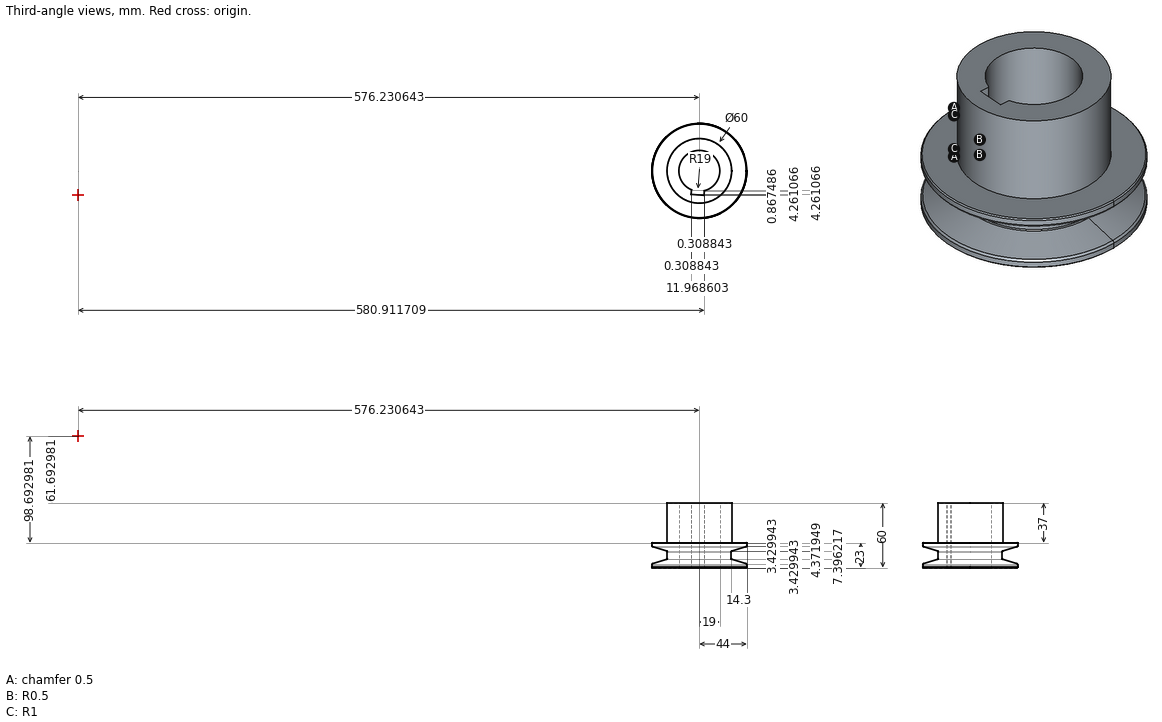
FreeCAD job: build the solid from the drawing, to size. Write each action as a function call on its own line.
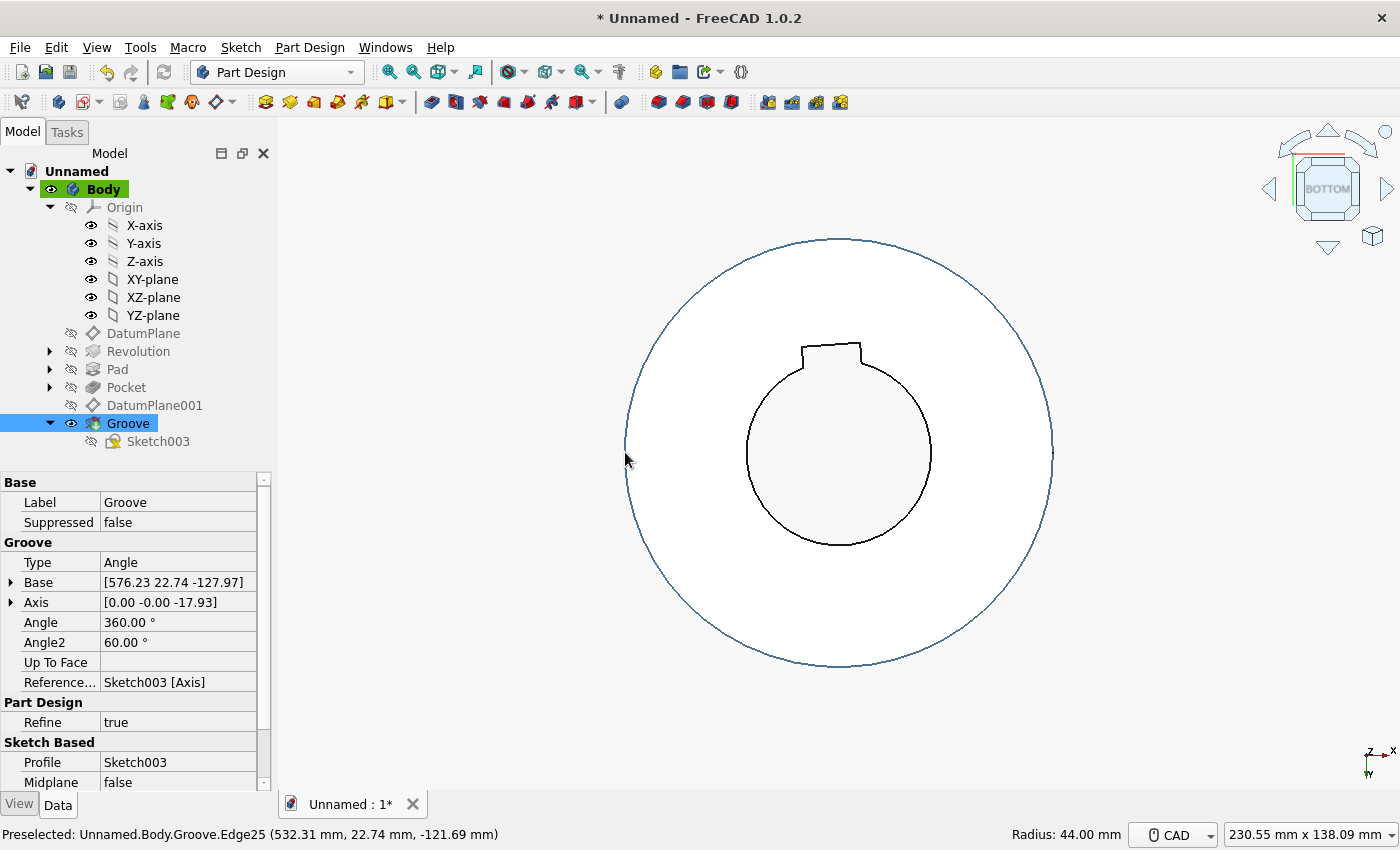
key(0)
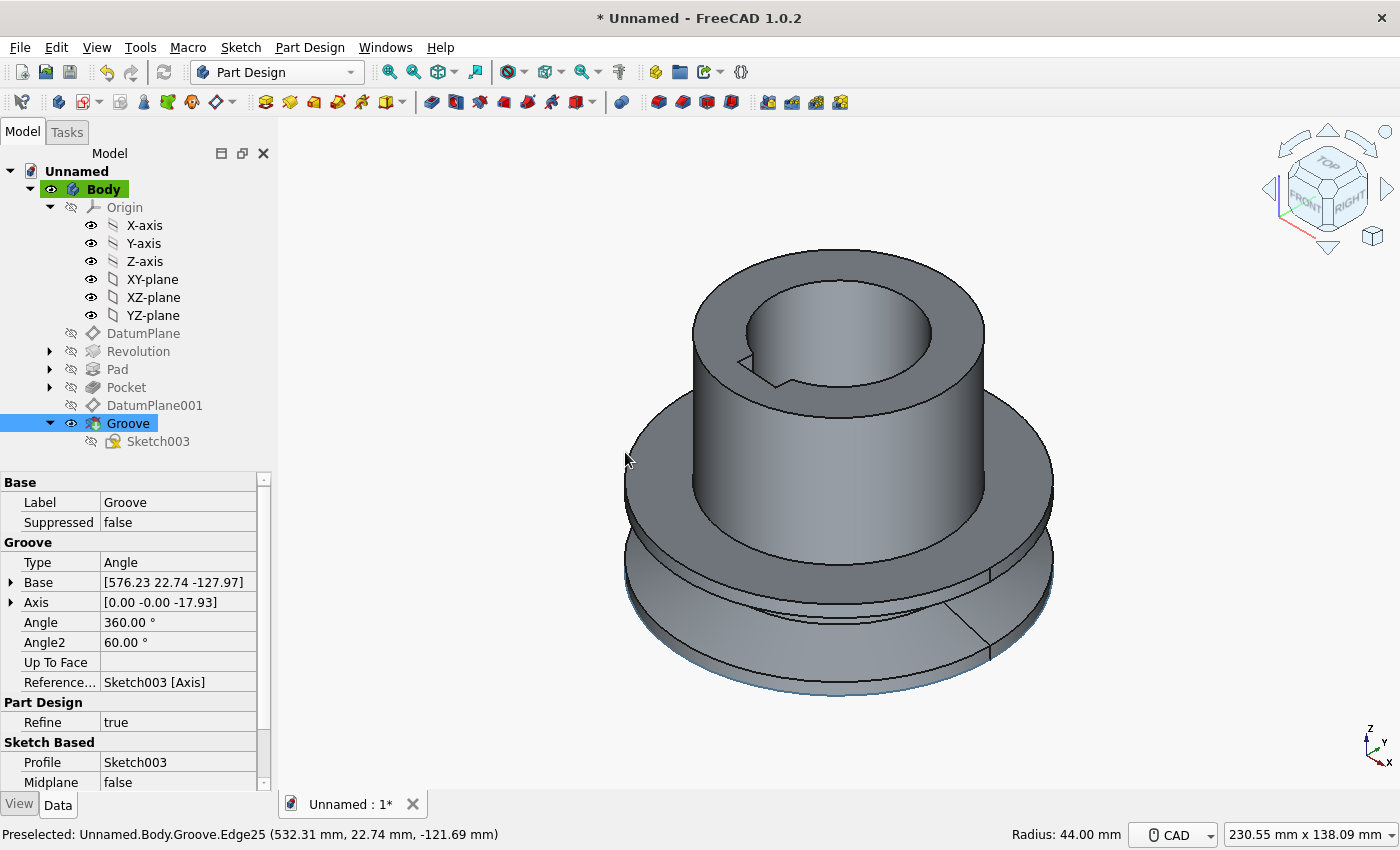
click(627, 460, ctrl)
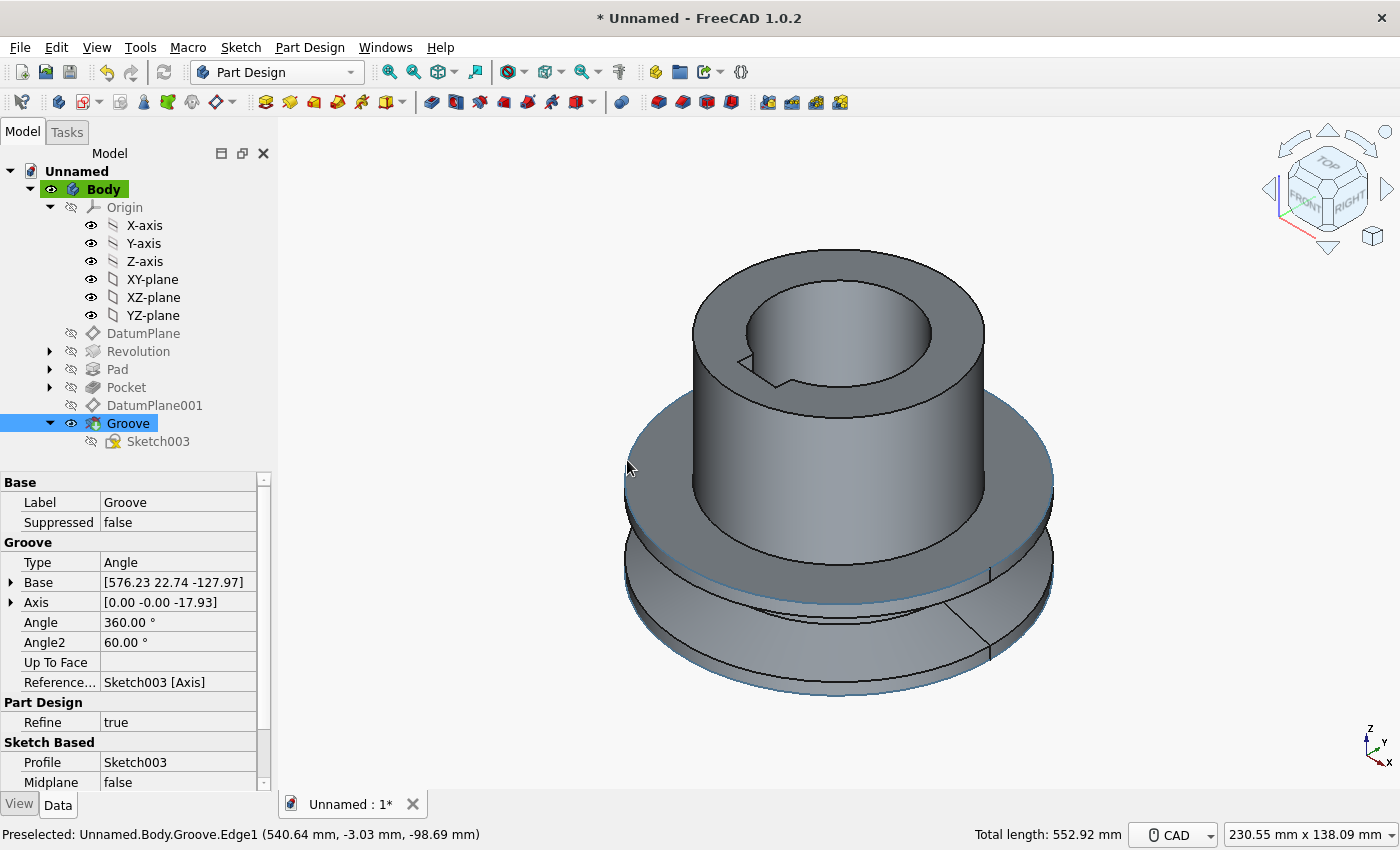
click(684, 102)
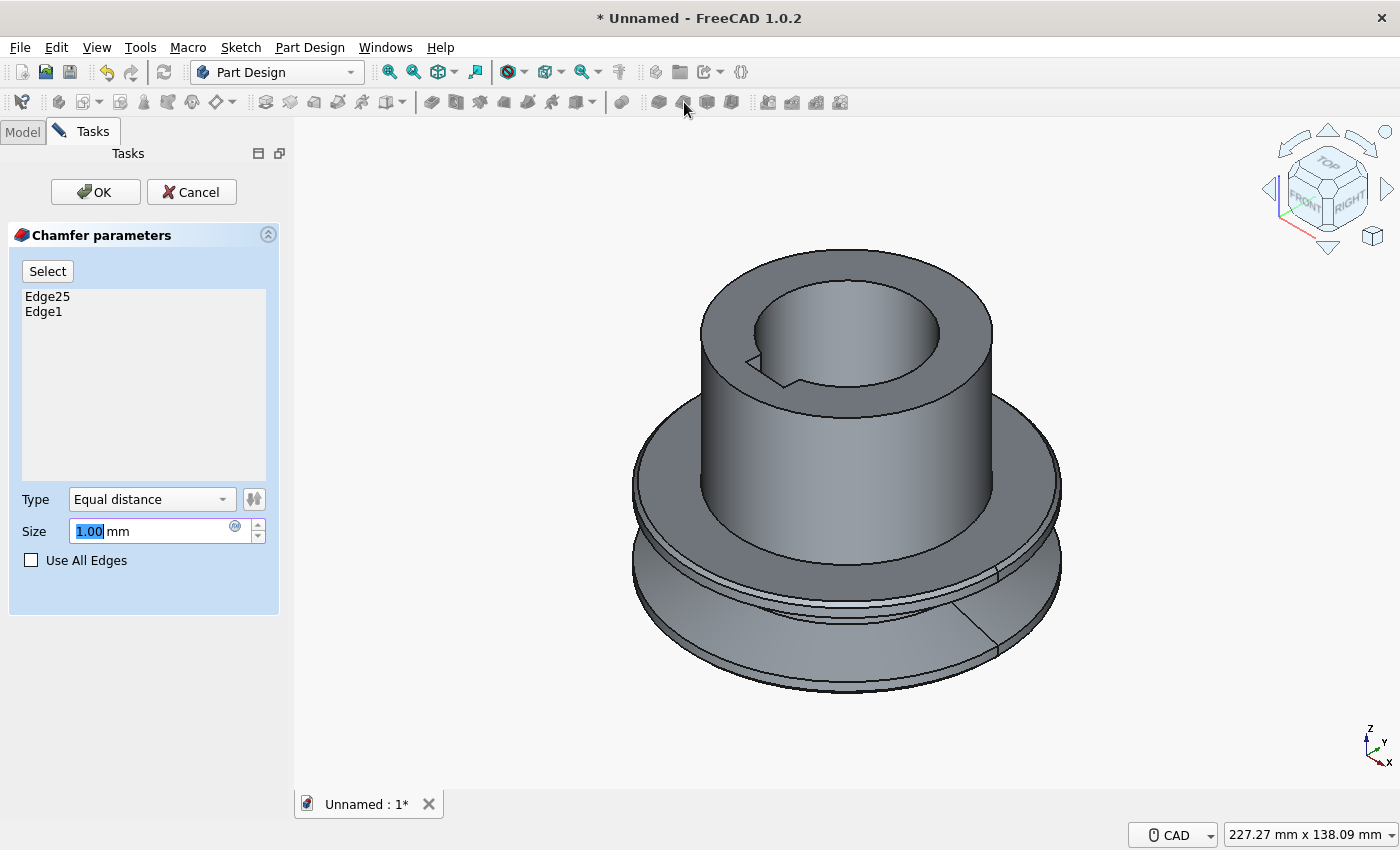
text(0.5)
key(Tab)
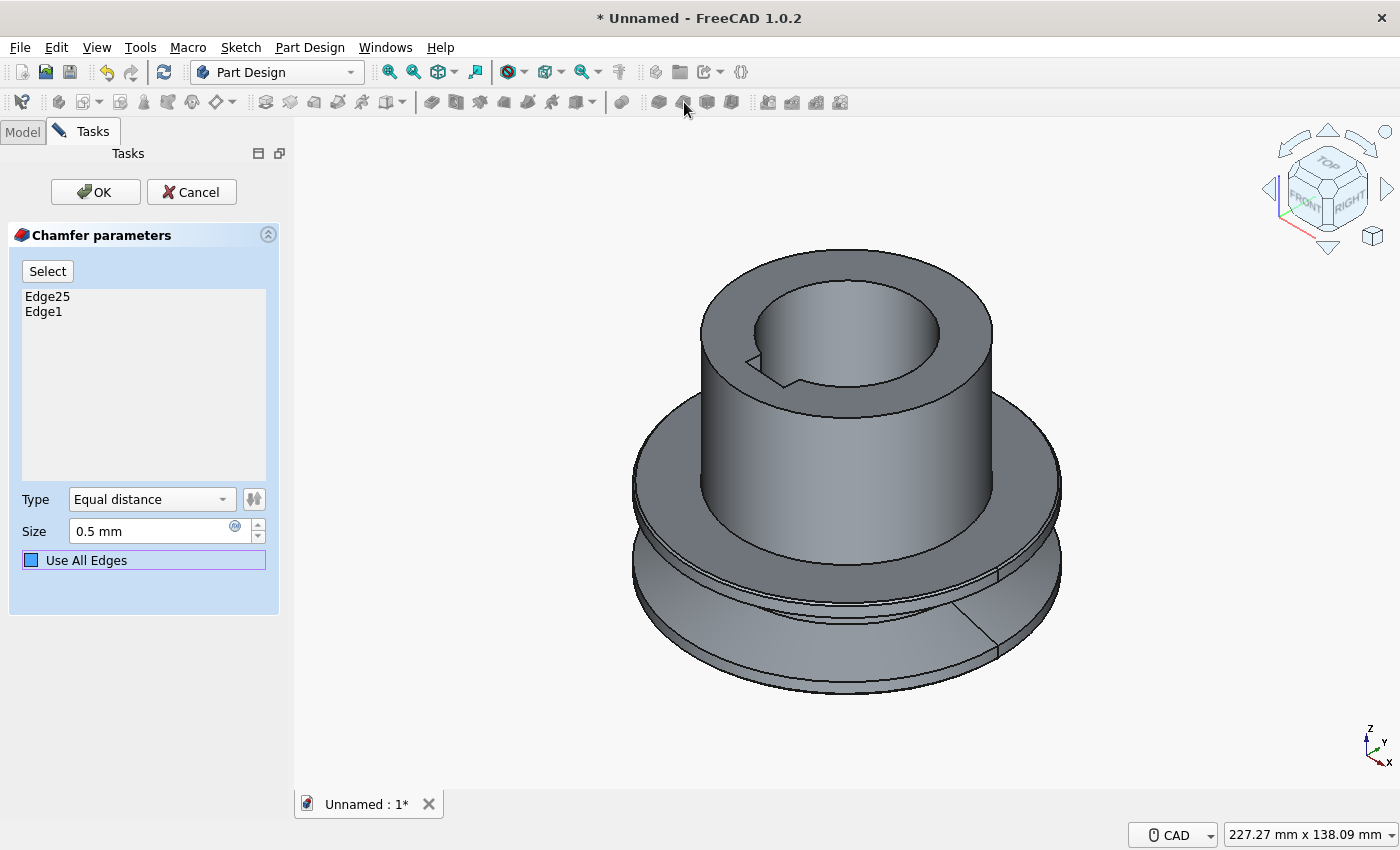
click(96, 192)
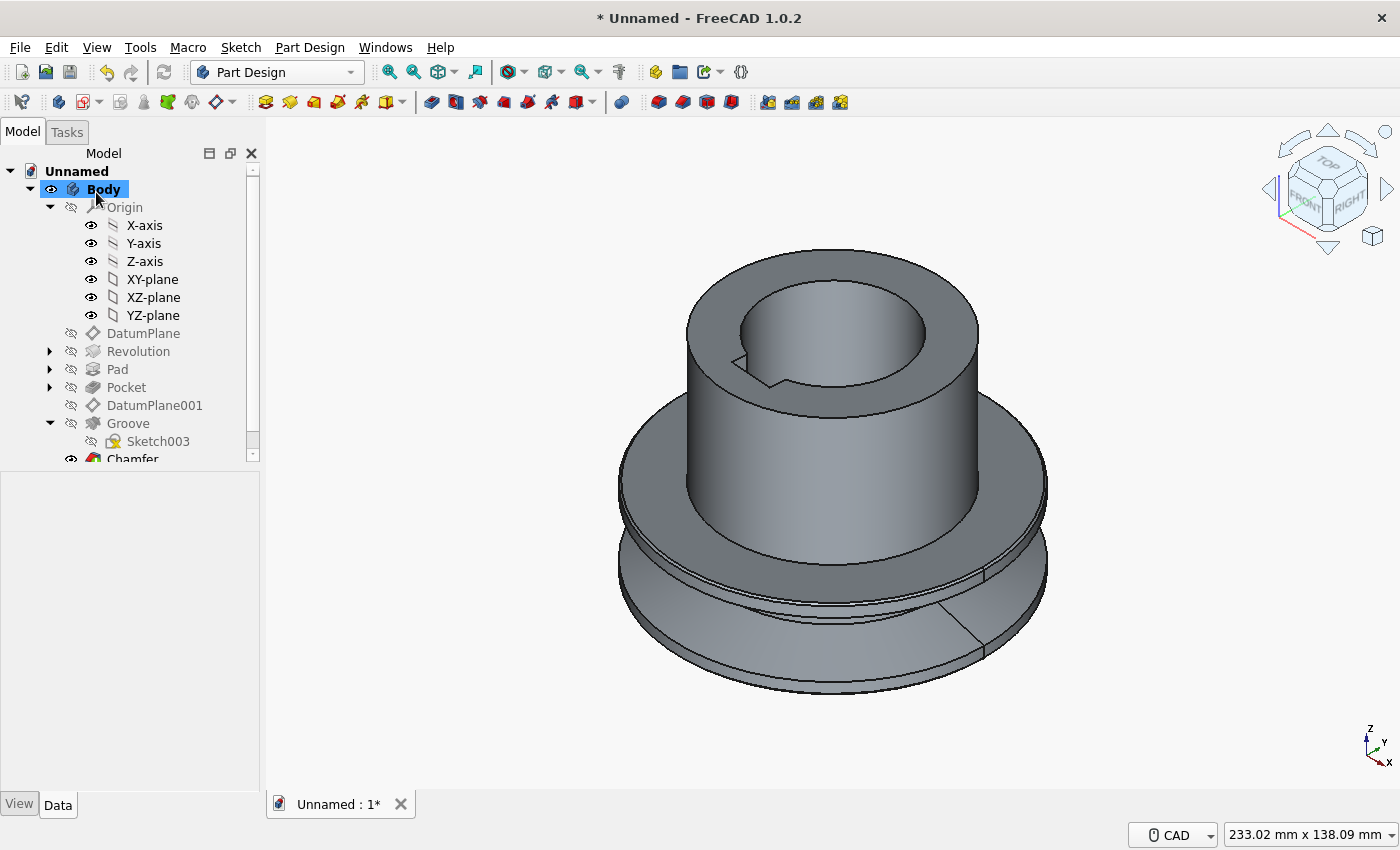
key(2)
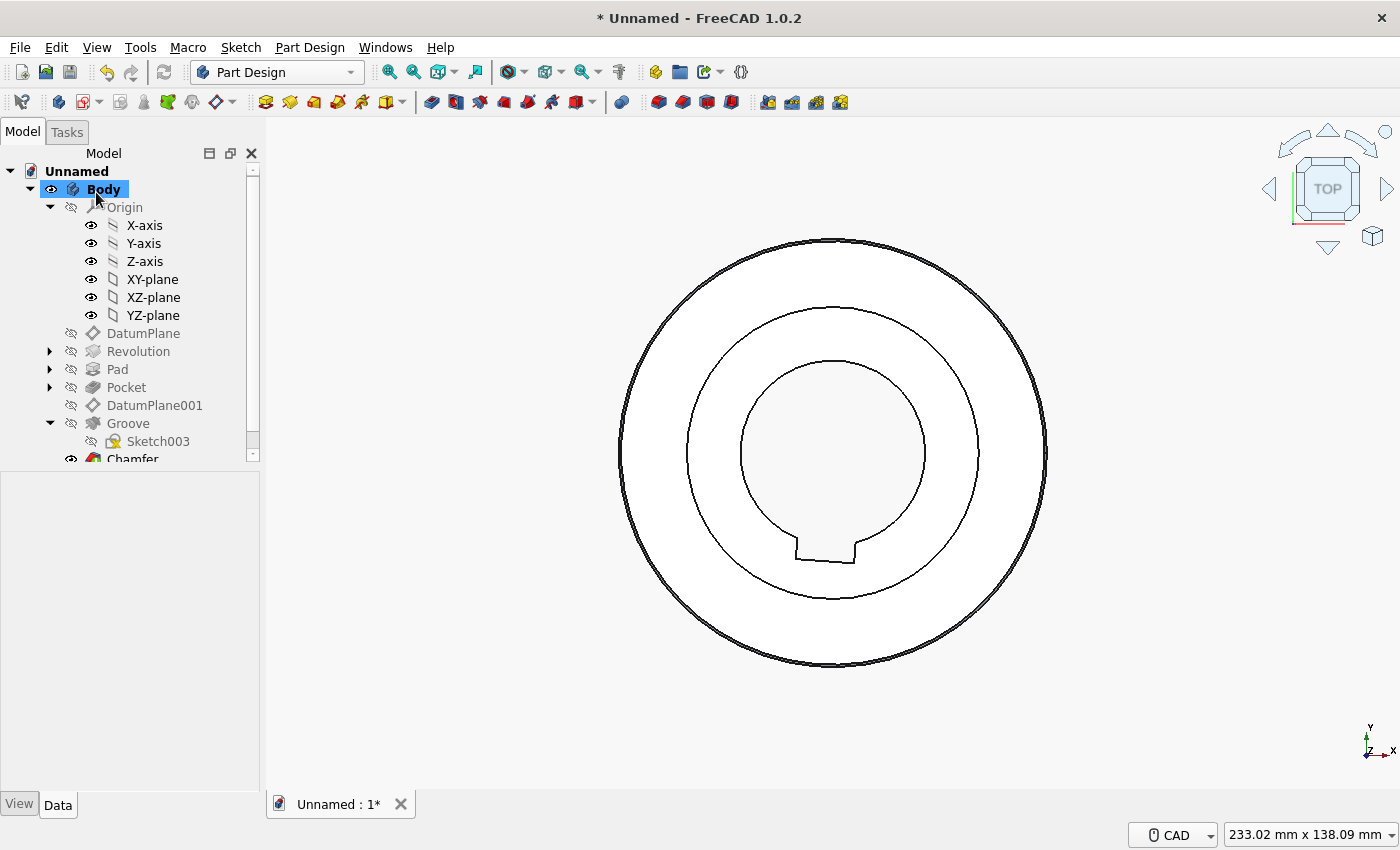
key(0)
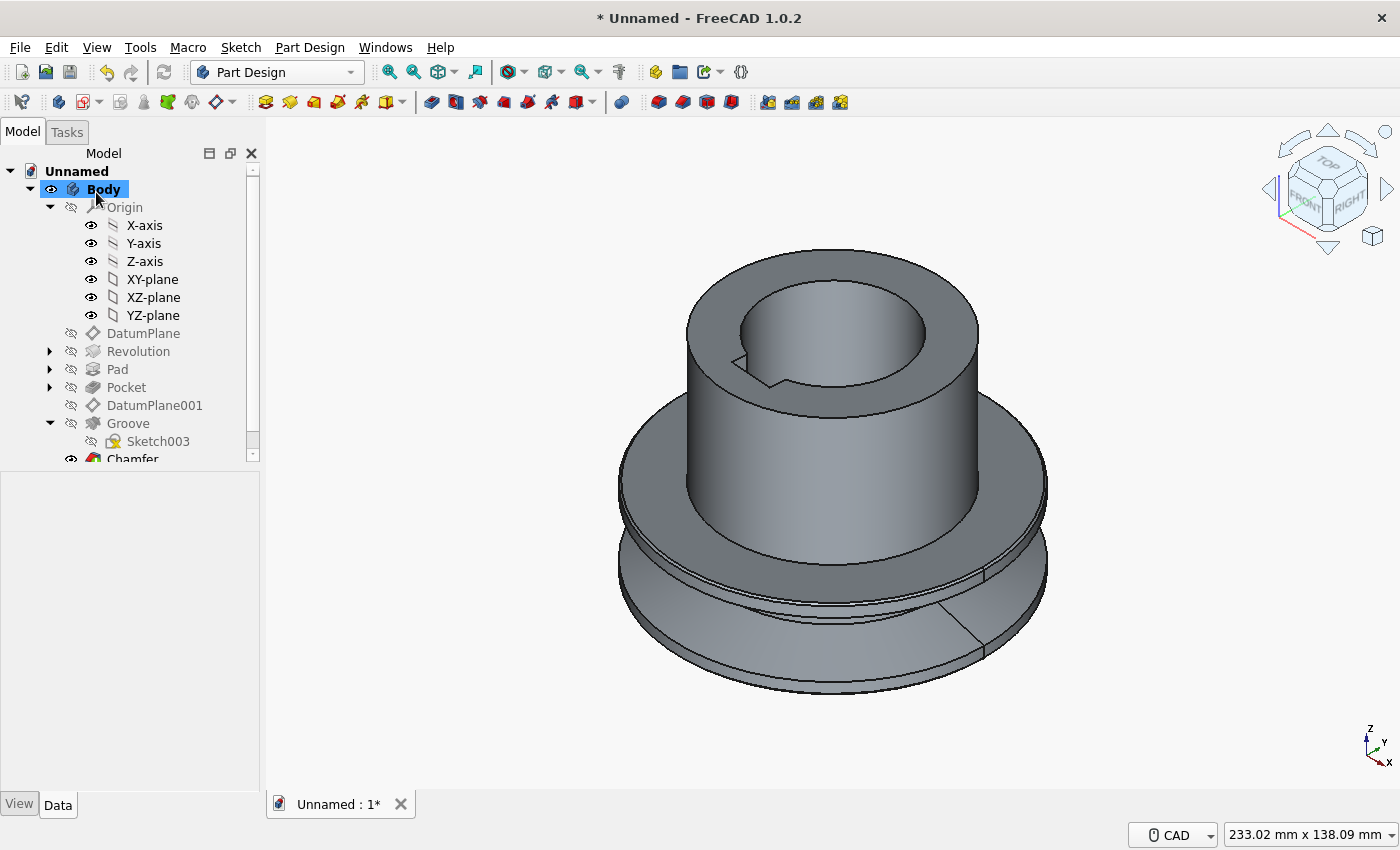
key(1)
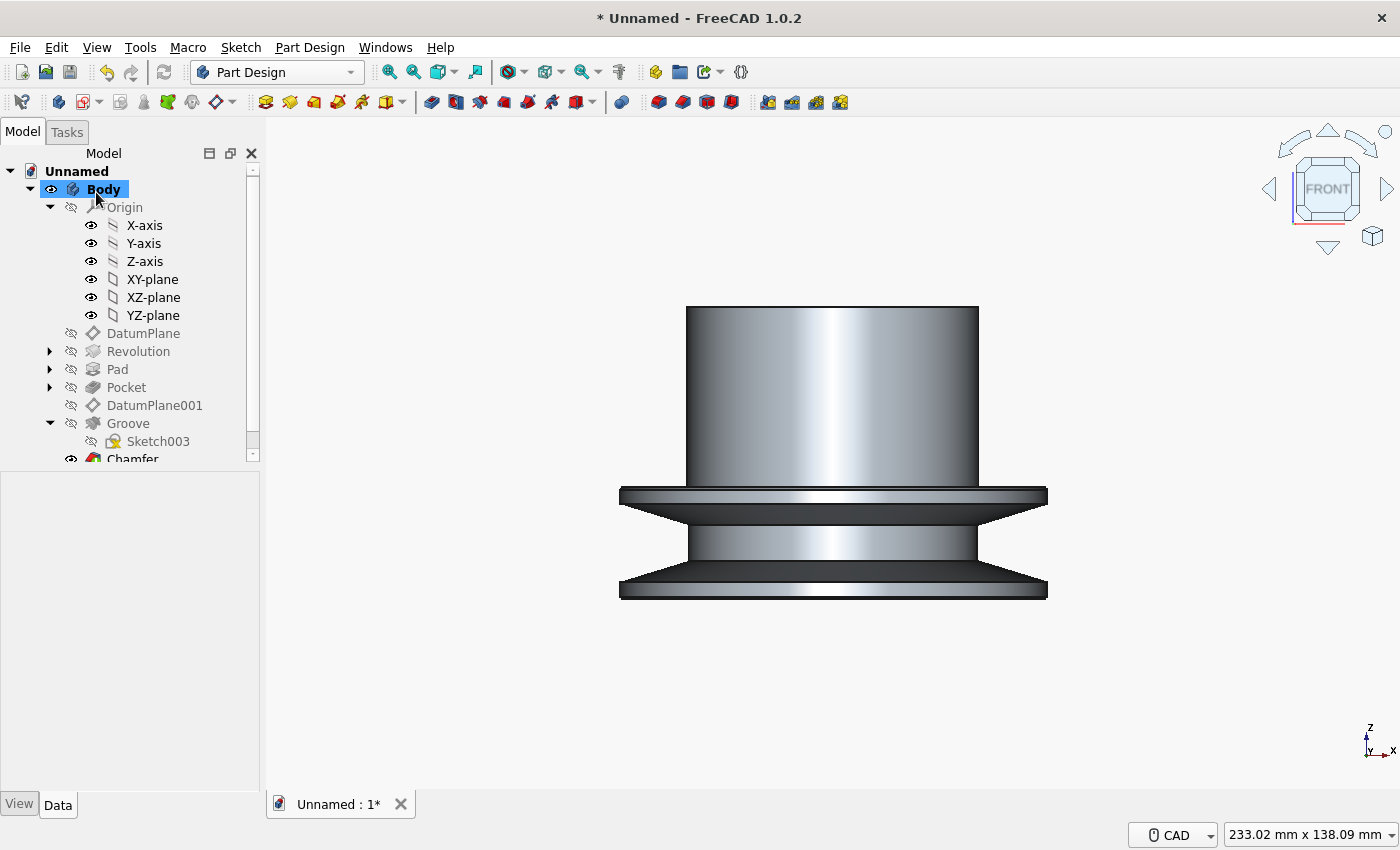
click(390, 72)